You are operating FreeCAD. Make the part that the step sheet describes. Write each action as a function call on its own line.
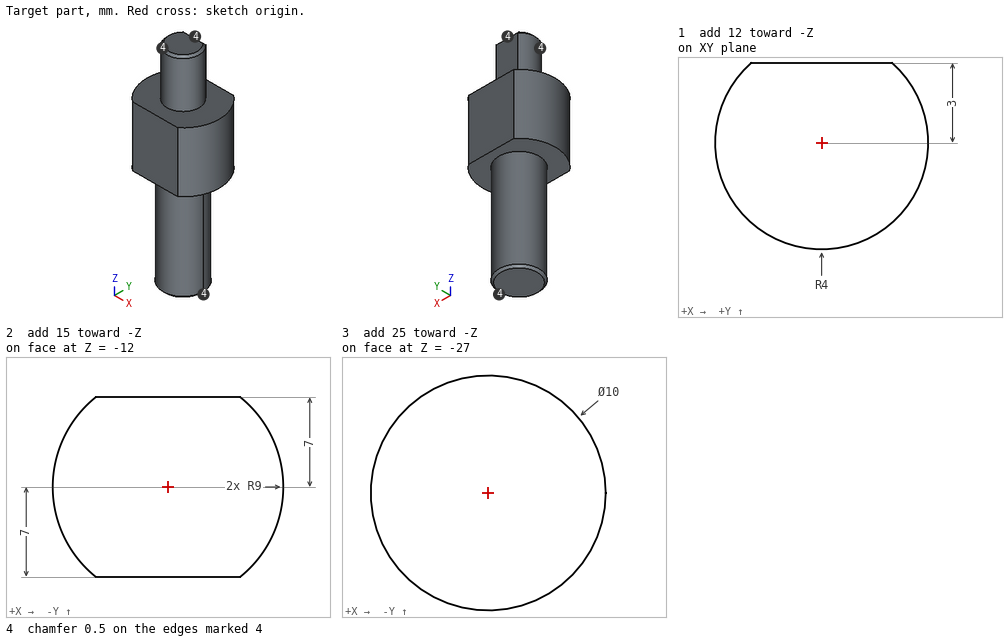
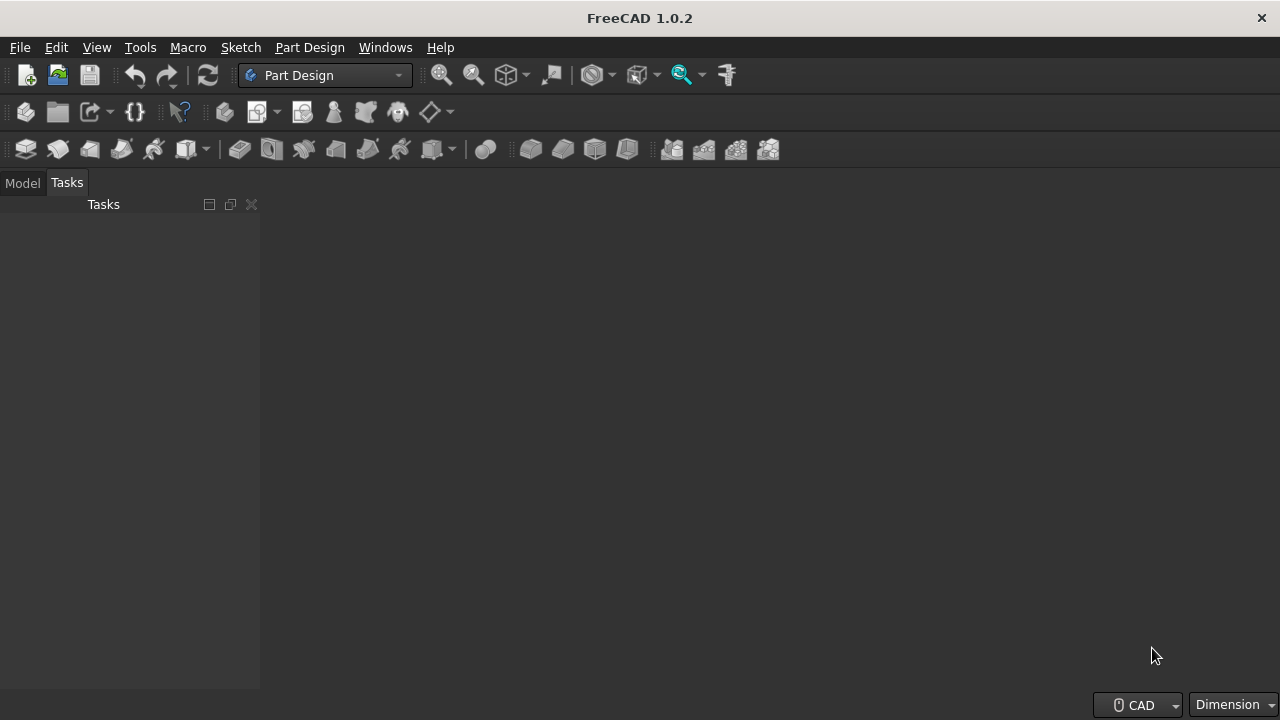
click(26, 76)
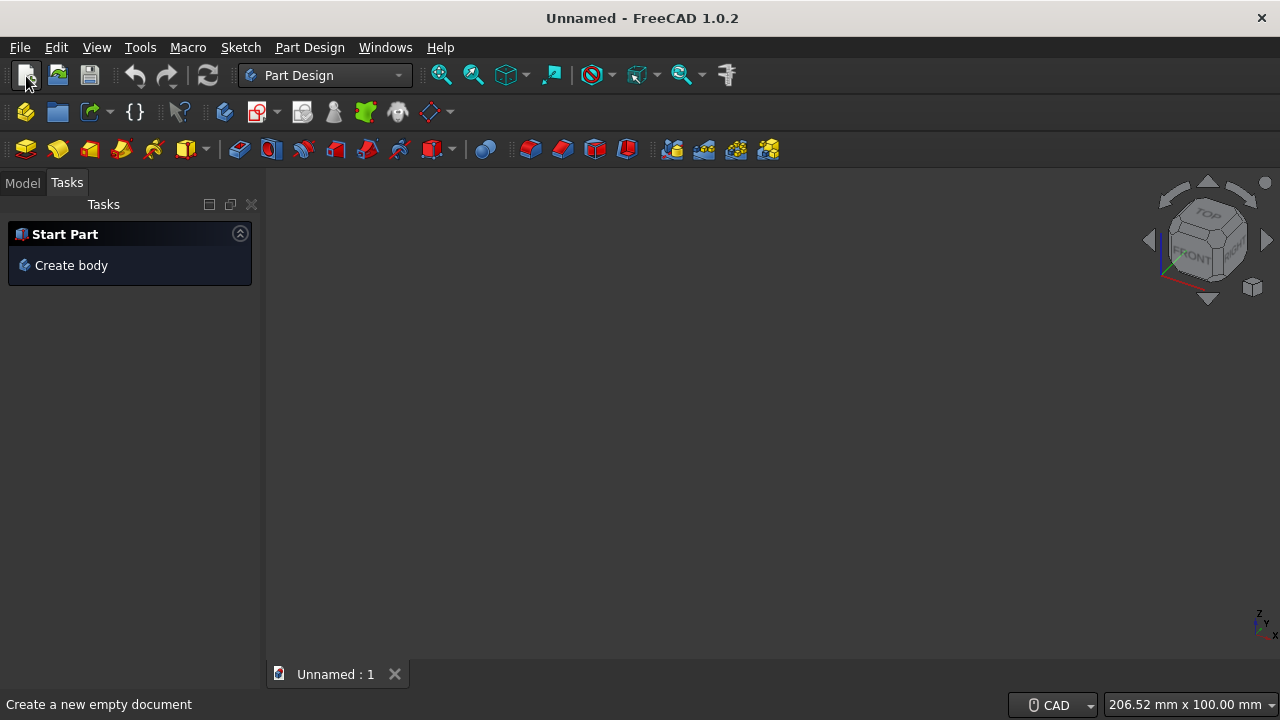
click(258, 112)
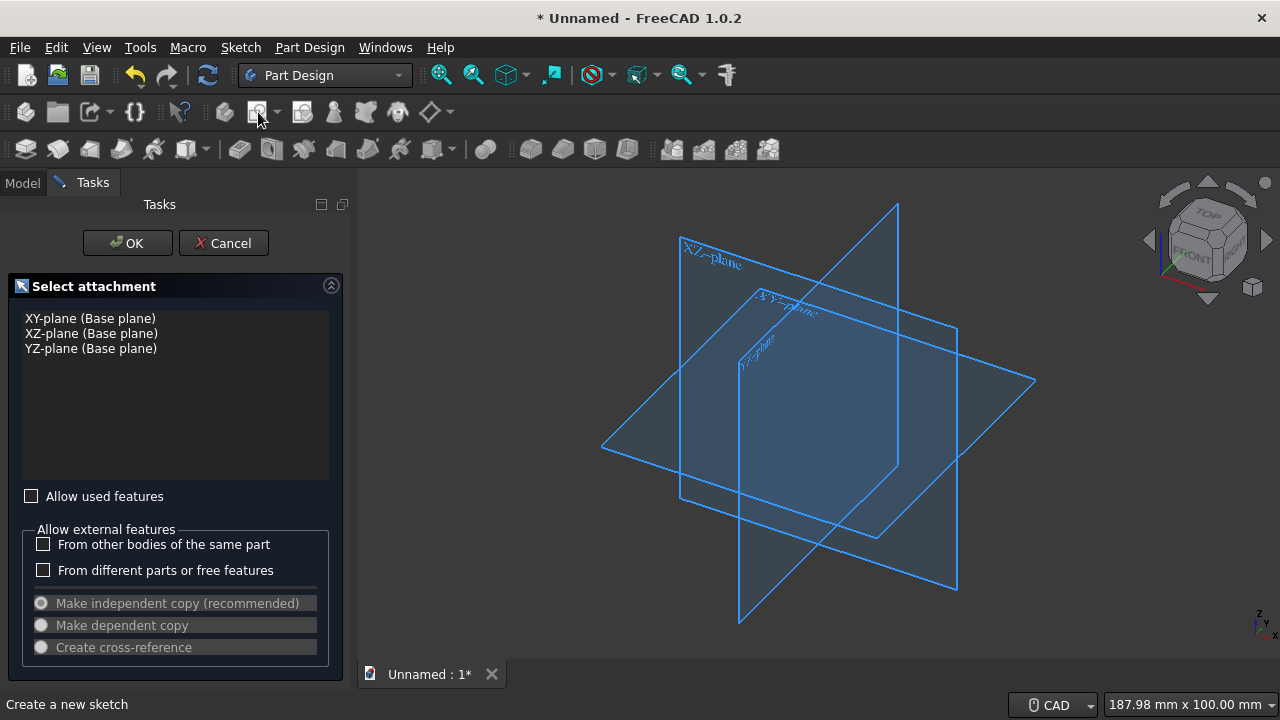
click(82, 318)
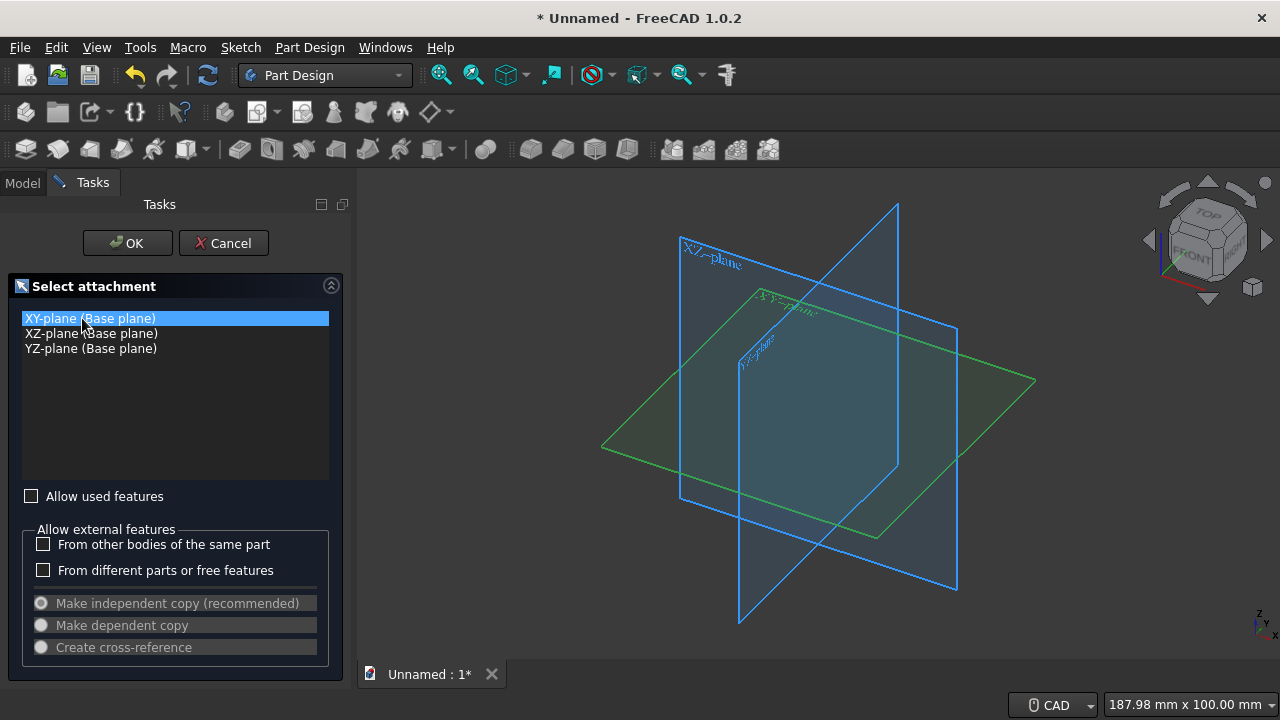
click(128, 243)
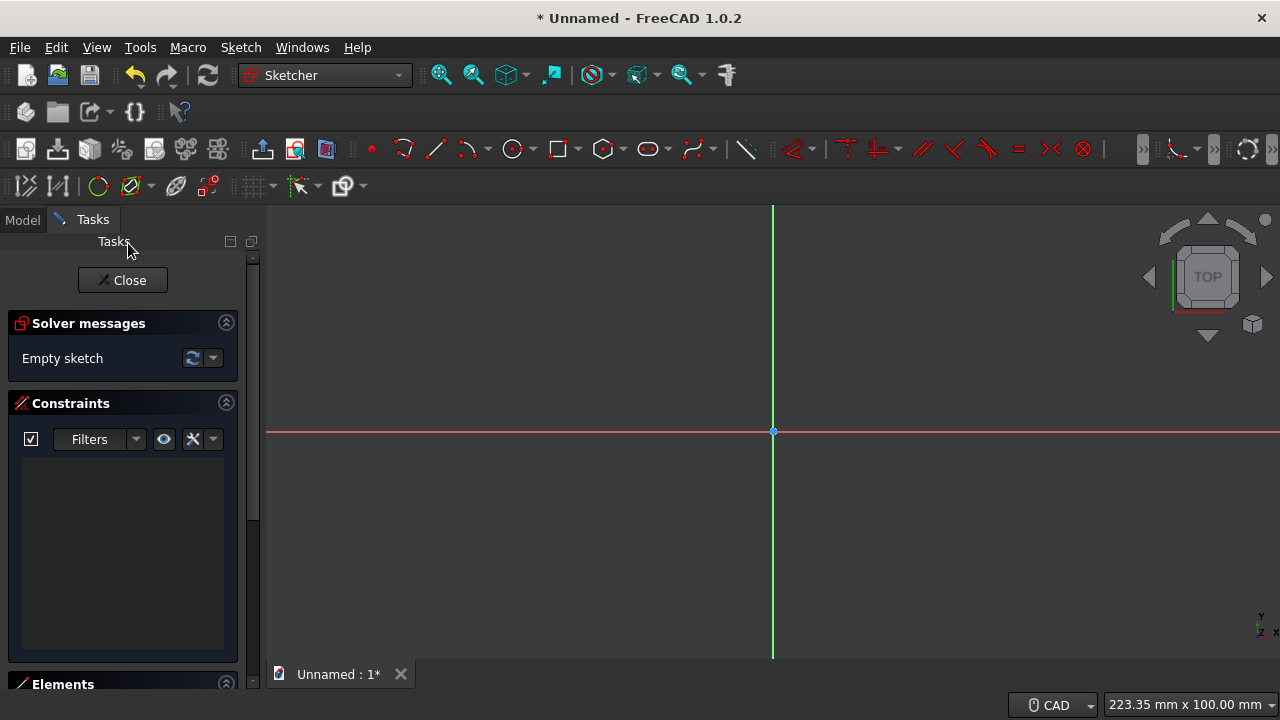
scroll(782, 435, up, 11)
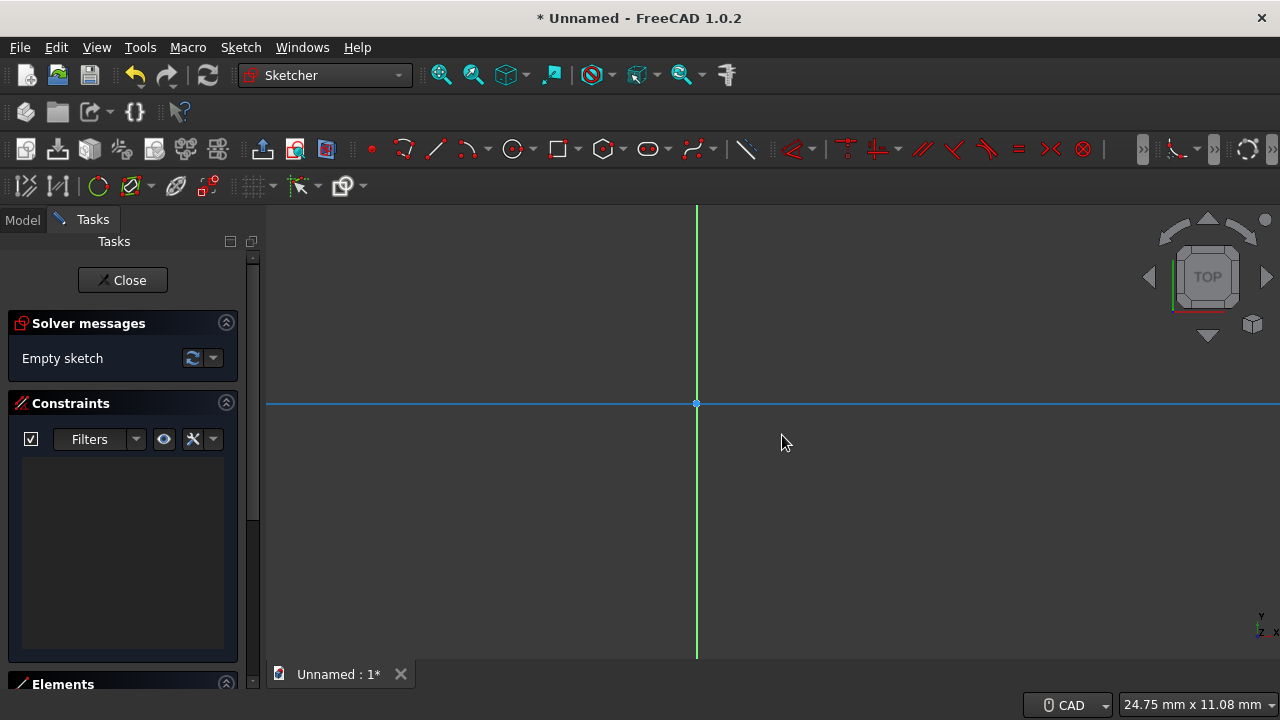
key(g)
key(l)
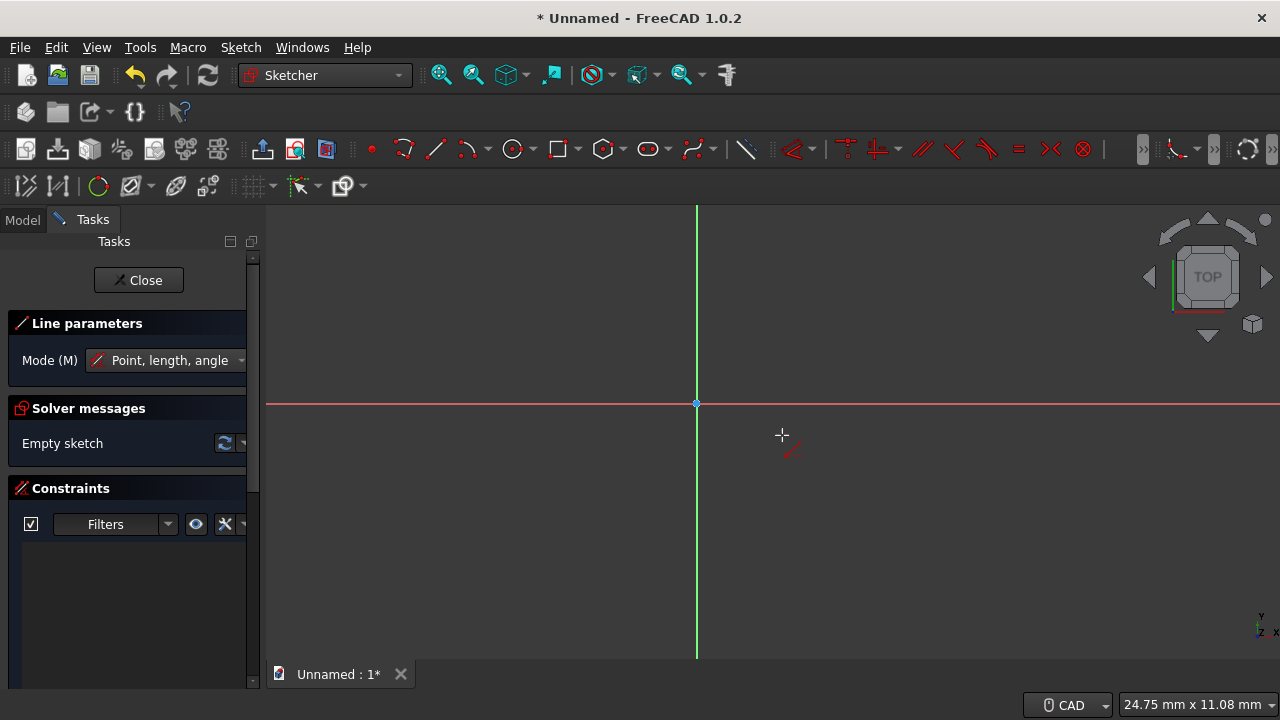
click(805, 281)
click(588, 281)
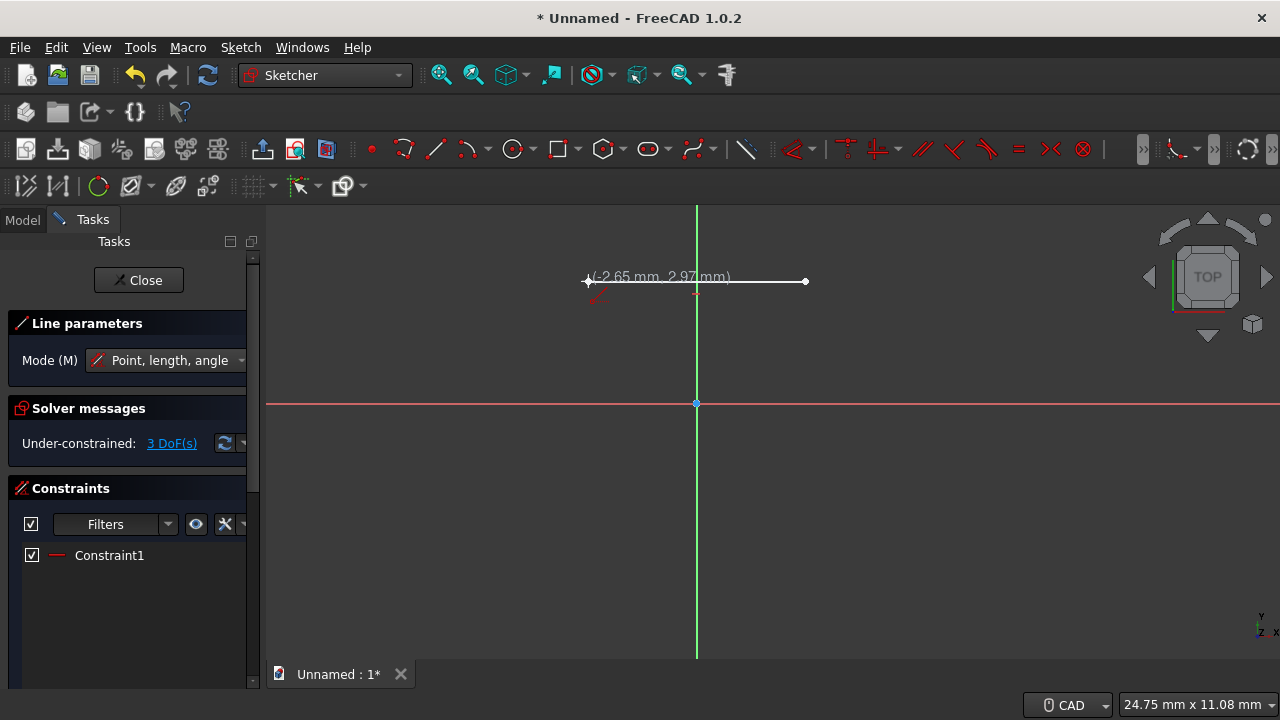
key(g)
key(3)
key(a)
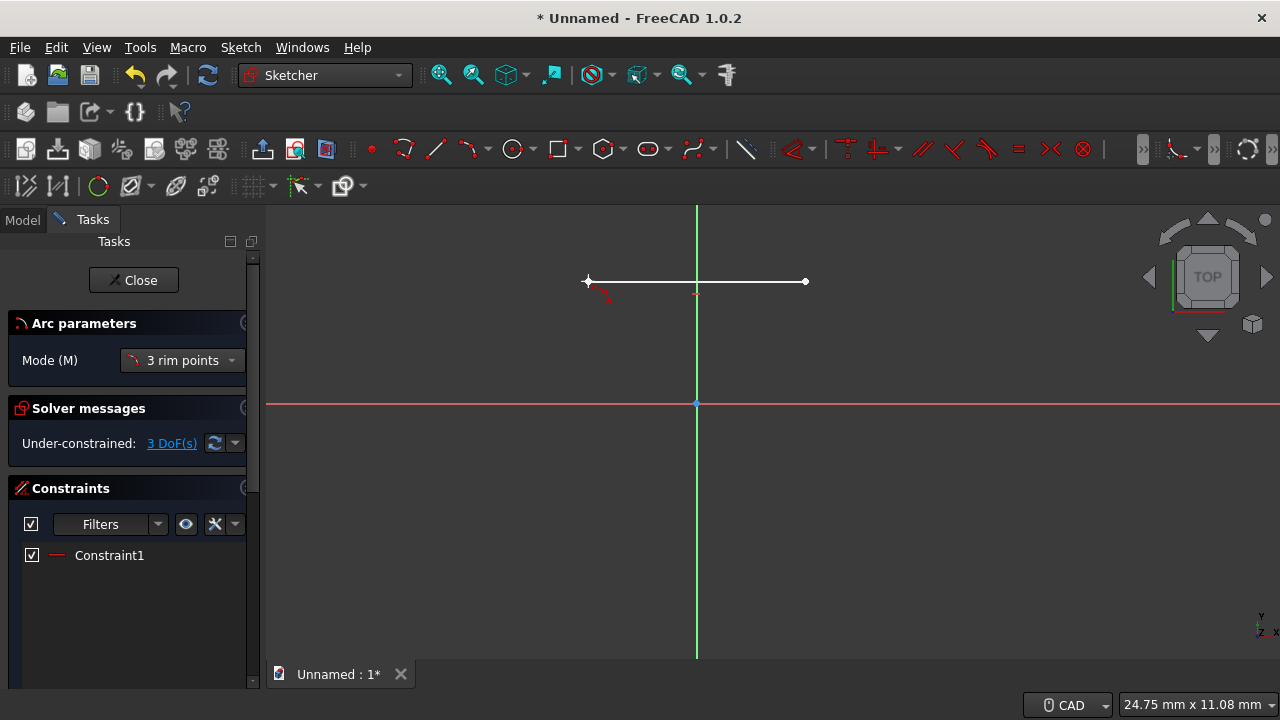
click(588, 282)
click(805, 282)
click(620, 549)
key(Escape)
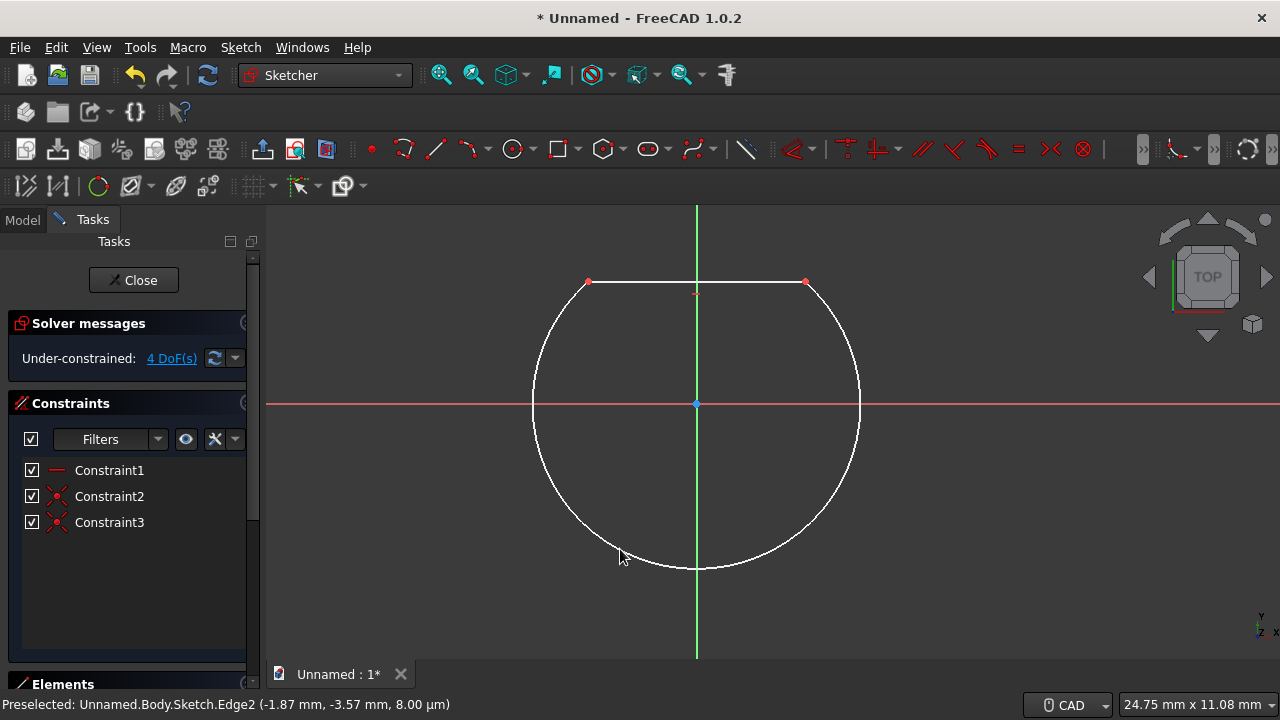
drag(686, 394, 707, 415)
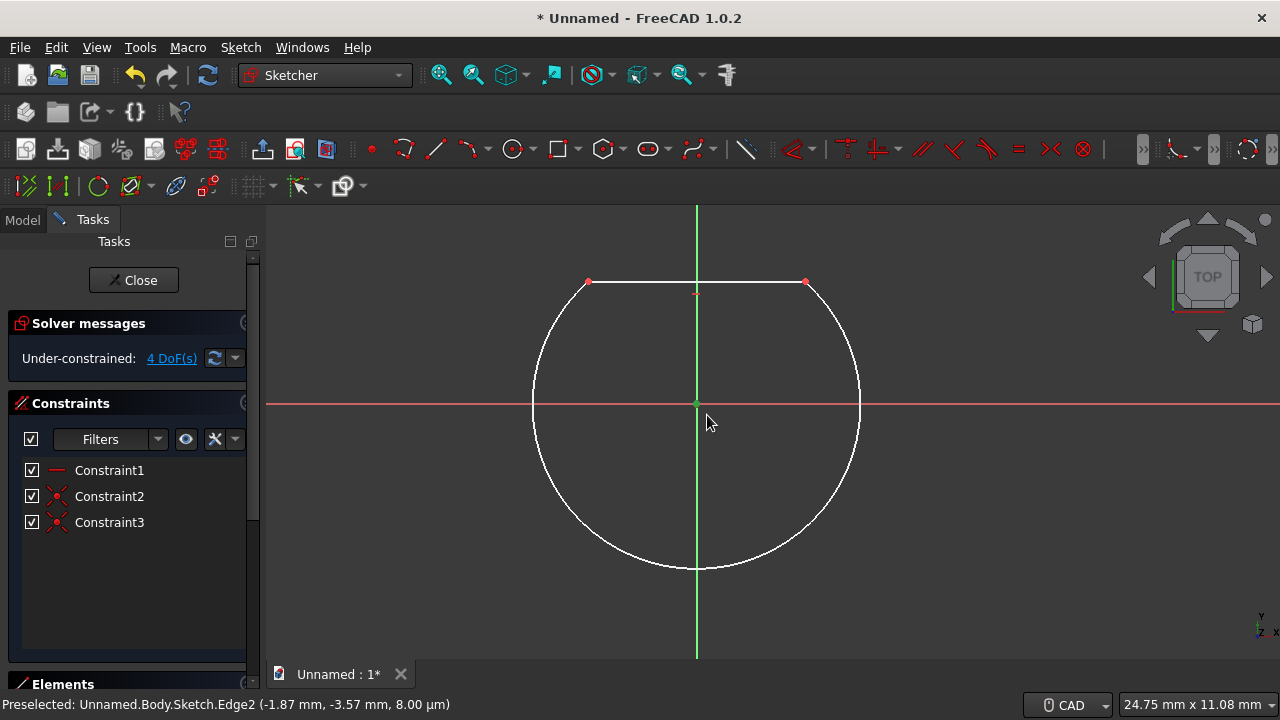
key(c)